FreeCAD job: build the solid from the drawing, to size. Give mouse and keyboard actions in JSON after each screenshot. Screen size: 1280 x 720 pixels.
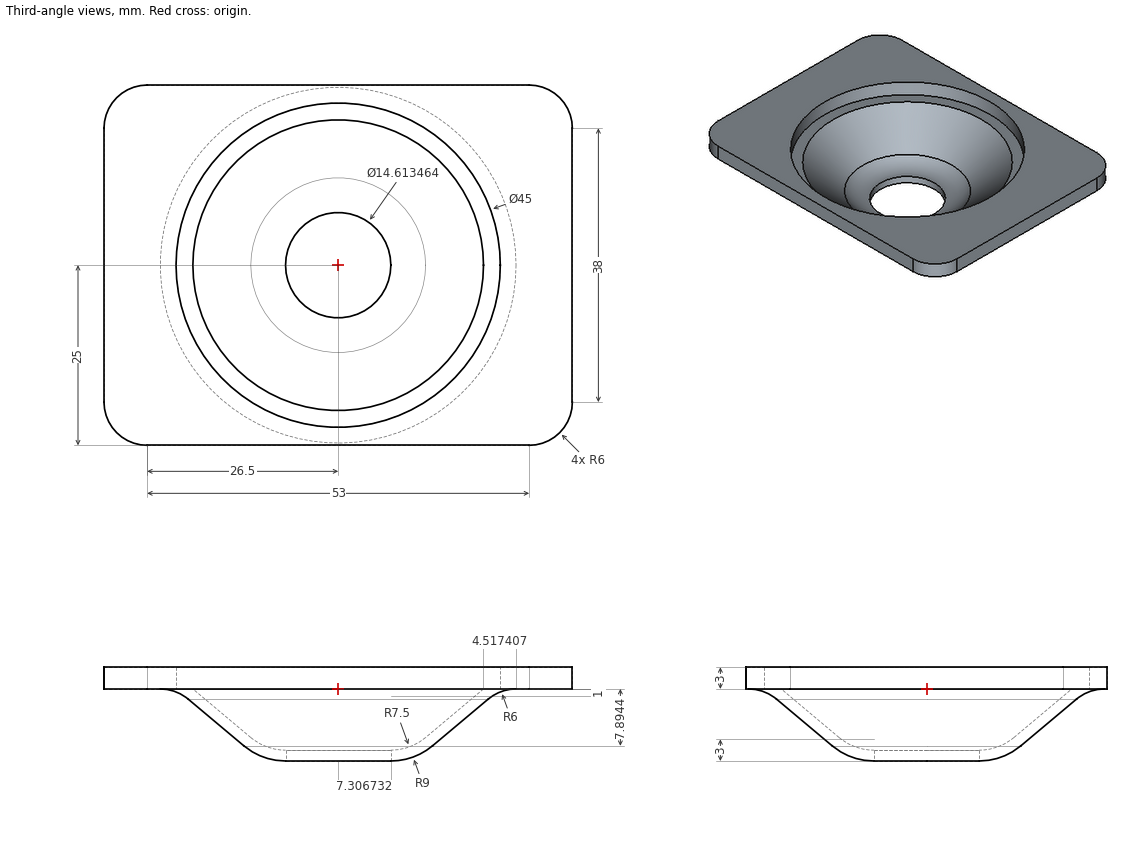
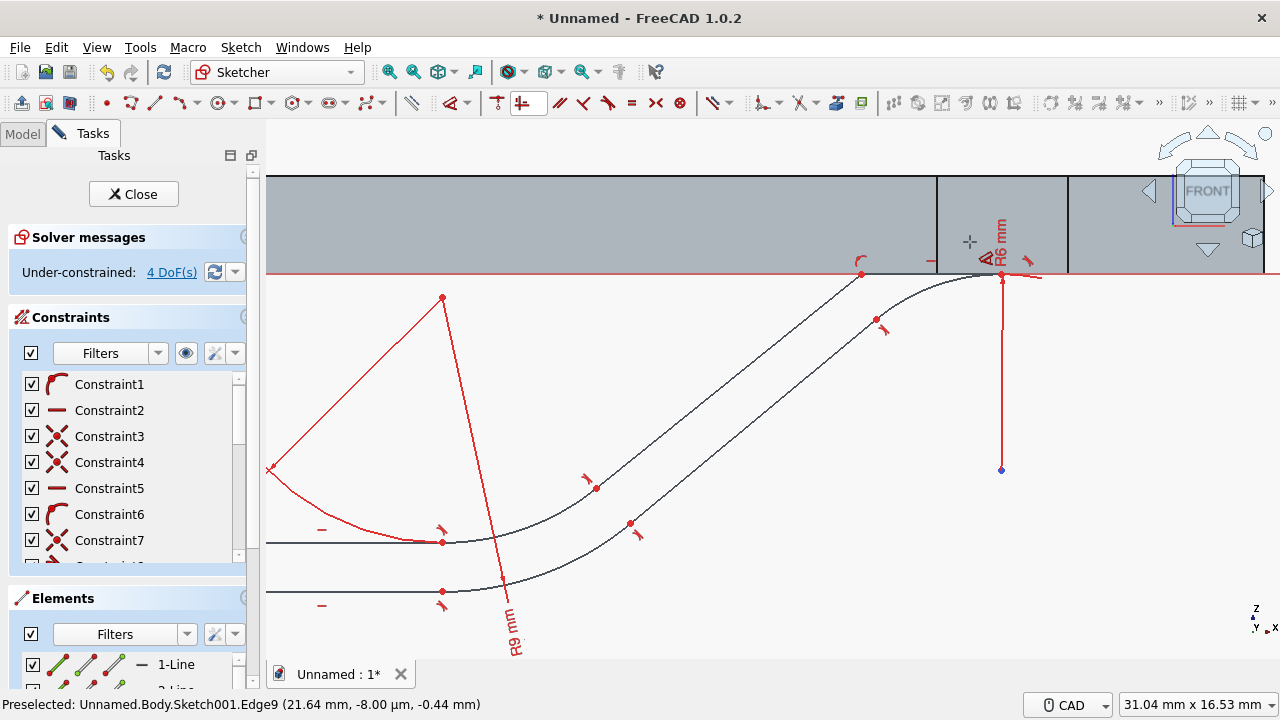
{"action": "left_click", "coordinate": [442, 298]}
{"action": "left_click", "coordinate": [476, 292]}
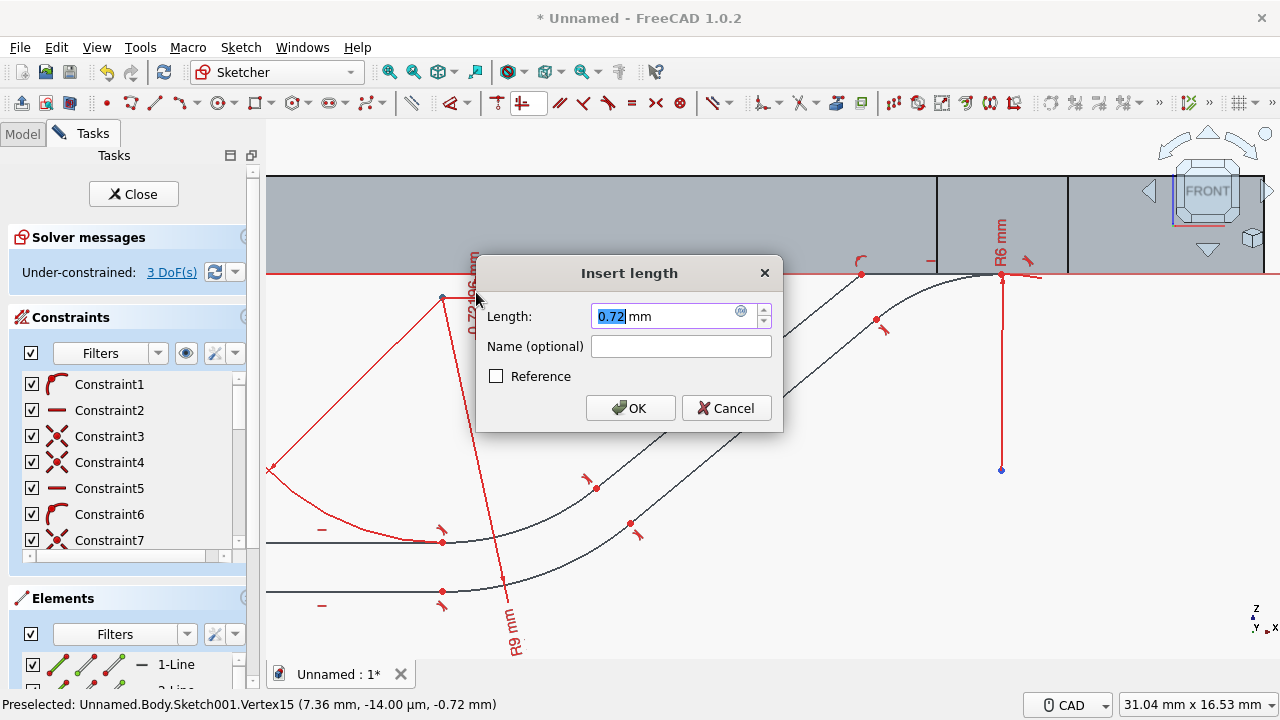
{"action": "type", "text": "1"}
{"action": "key", "text": "Return"}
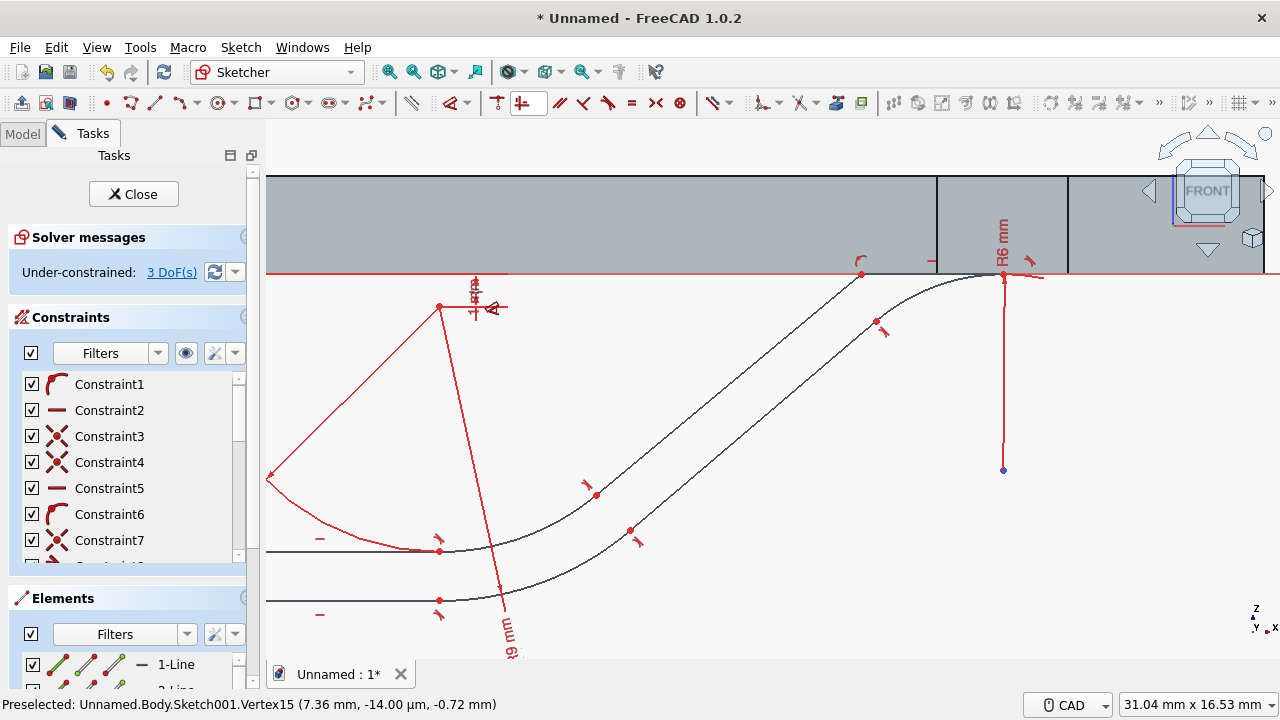
{"action": "left_click", "coordinate": [630, 531]}
{"action": "left_click", "coordinate": [664, 403]}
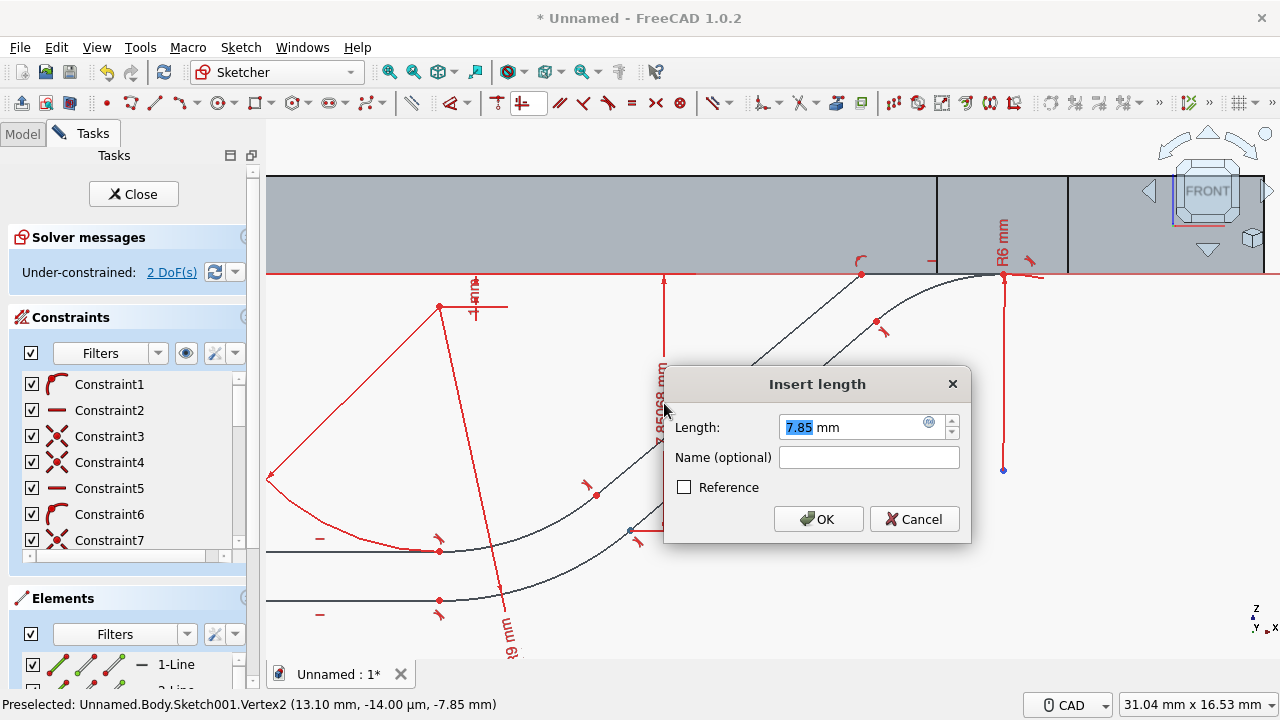
{"action": "type", "text": "7.8944"}
{"action": "key", "text": "Return"}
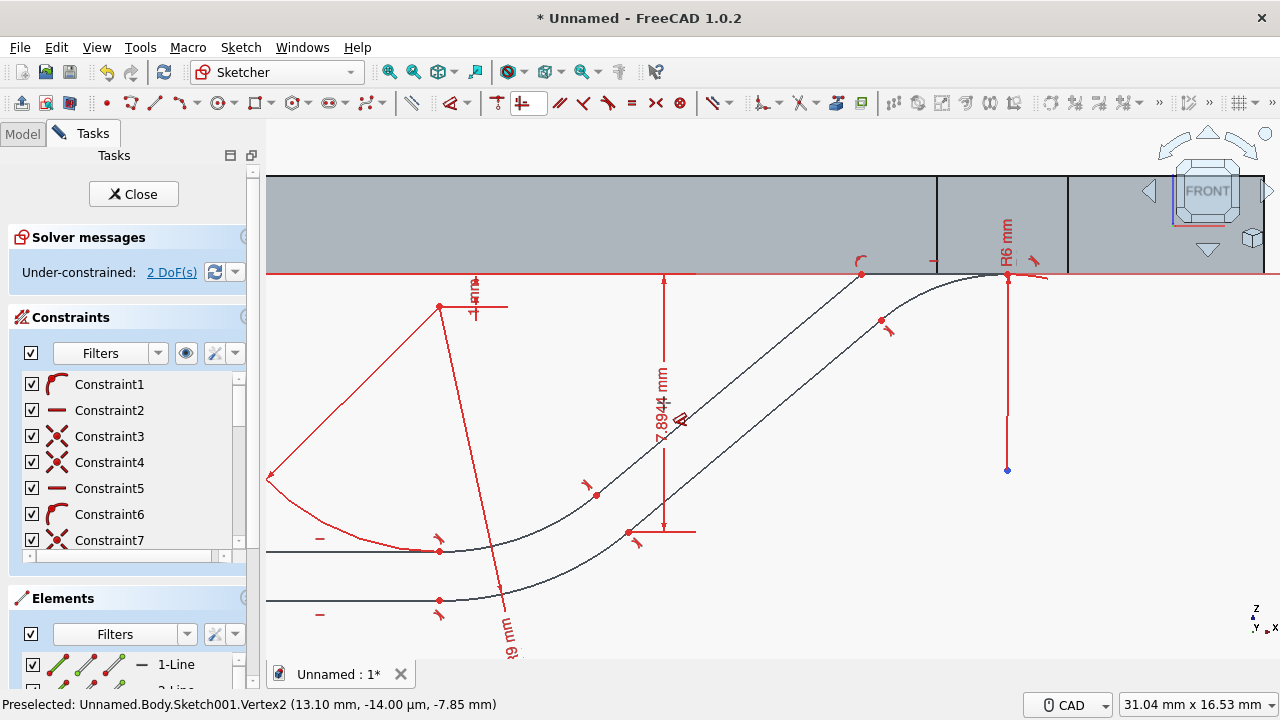
{"action": "left_click", "coordinate": [368, 601]}
{"action": "left_click", "coordinate": [367, 567]}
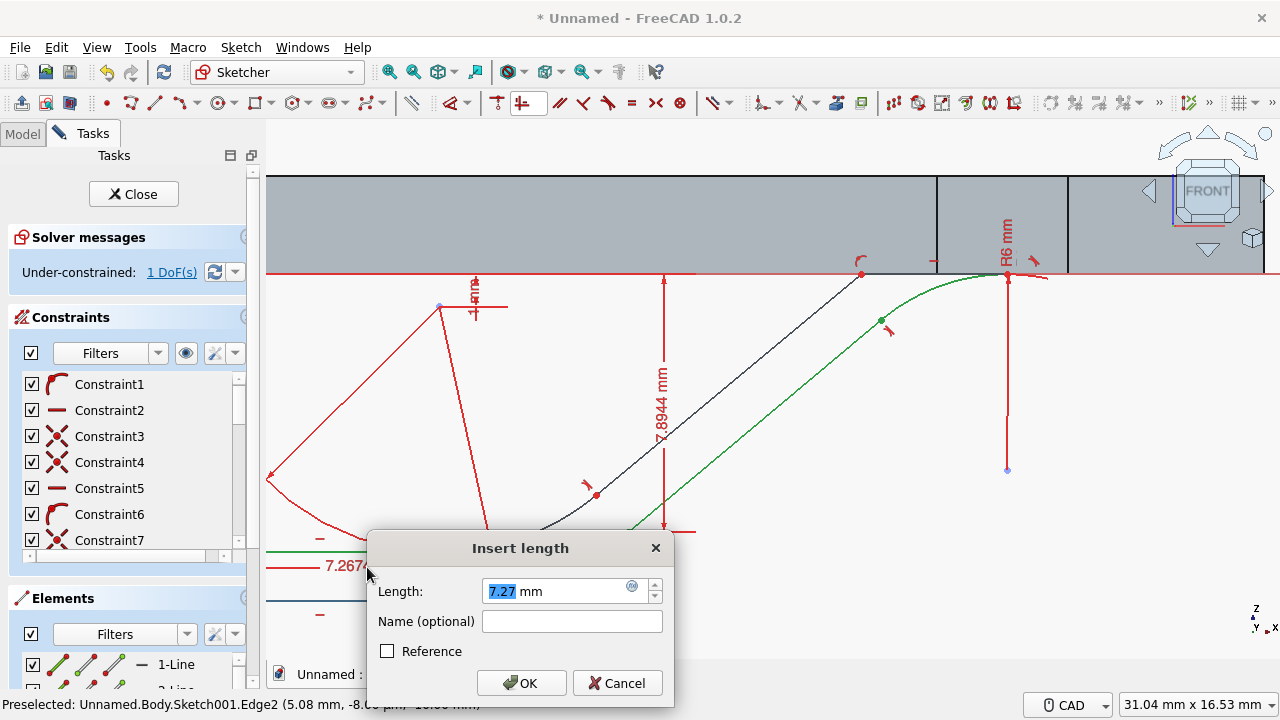
{"action": "type", "text": "7.306732"}
{"action": "key", "text": "Return"}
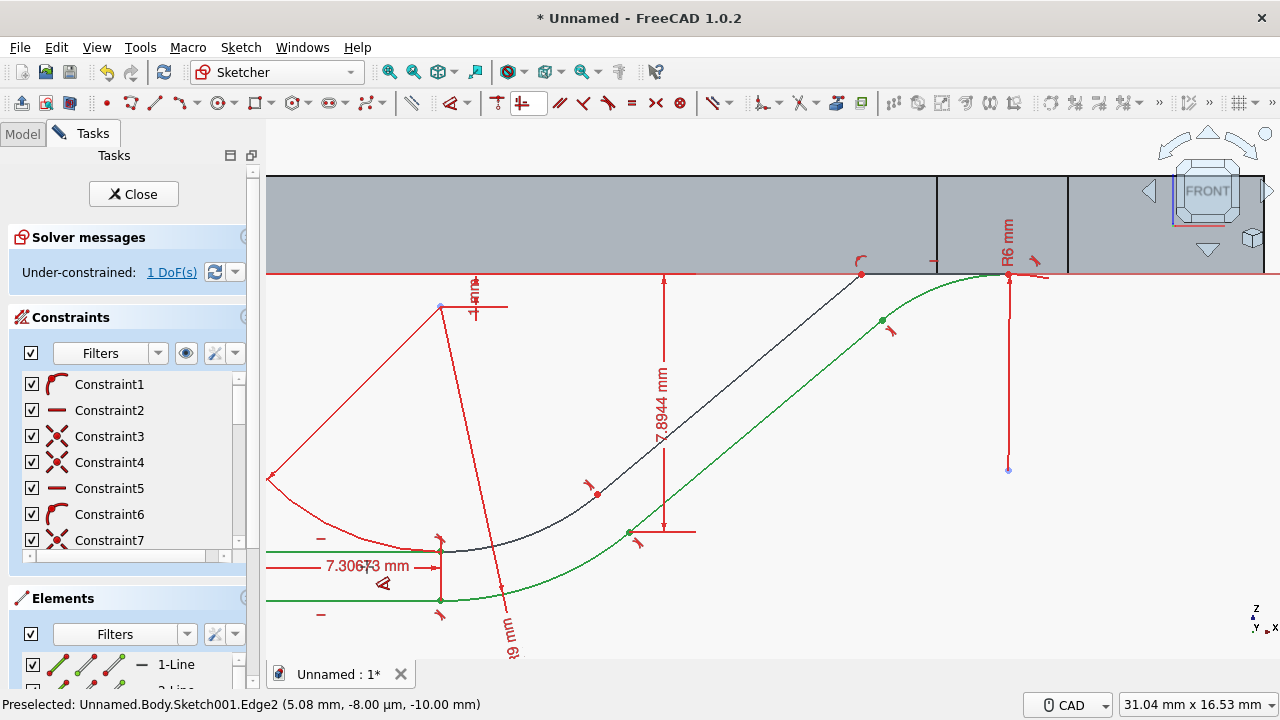
{"action": "left_click", "coordinate": [906, 274]}
{"action": "left_click", "coordinate": [884, 240]}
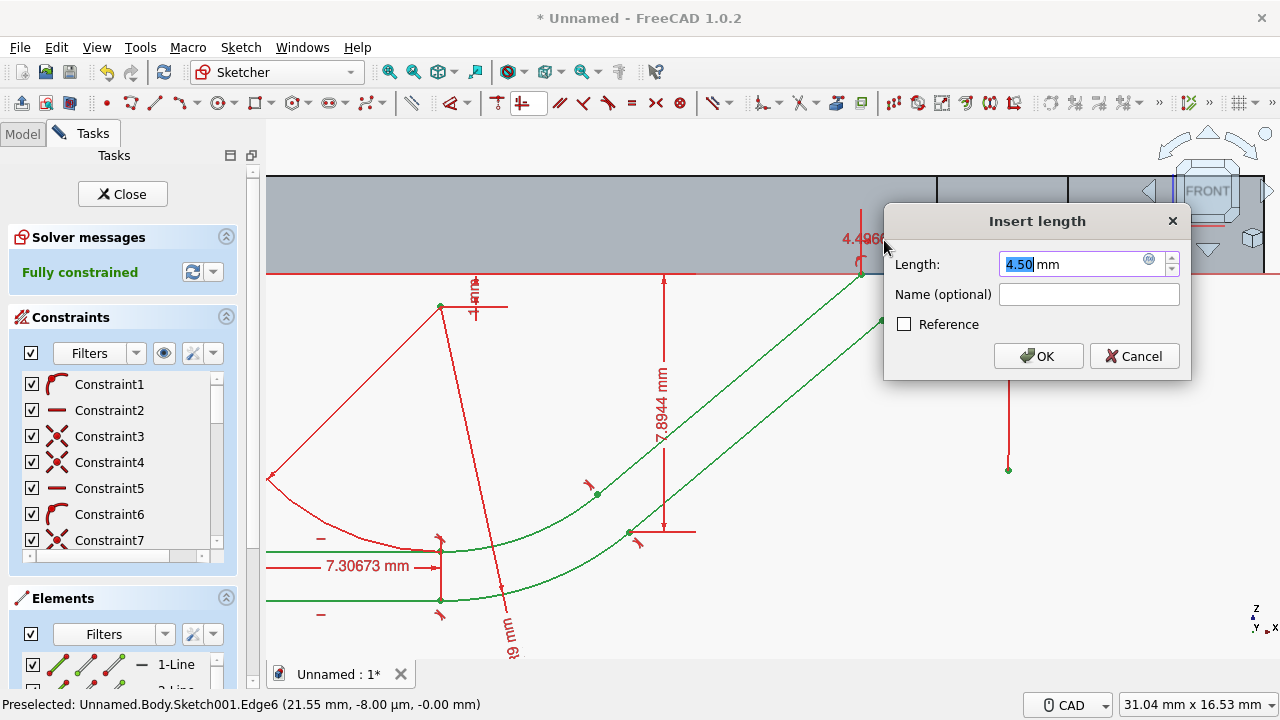
{"action": "type", "text": "4.517407"}
{"action": "key", "text": "Return"}
{"action": "key", "text": "Escape"}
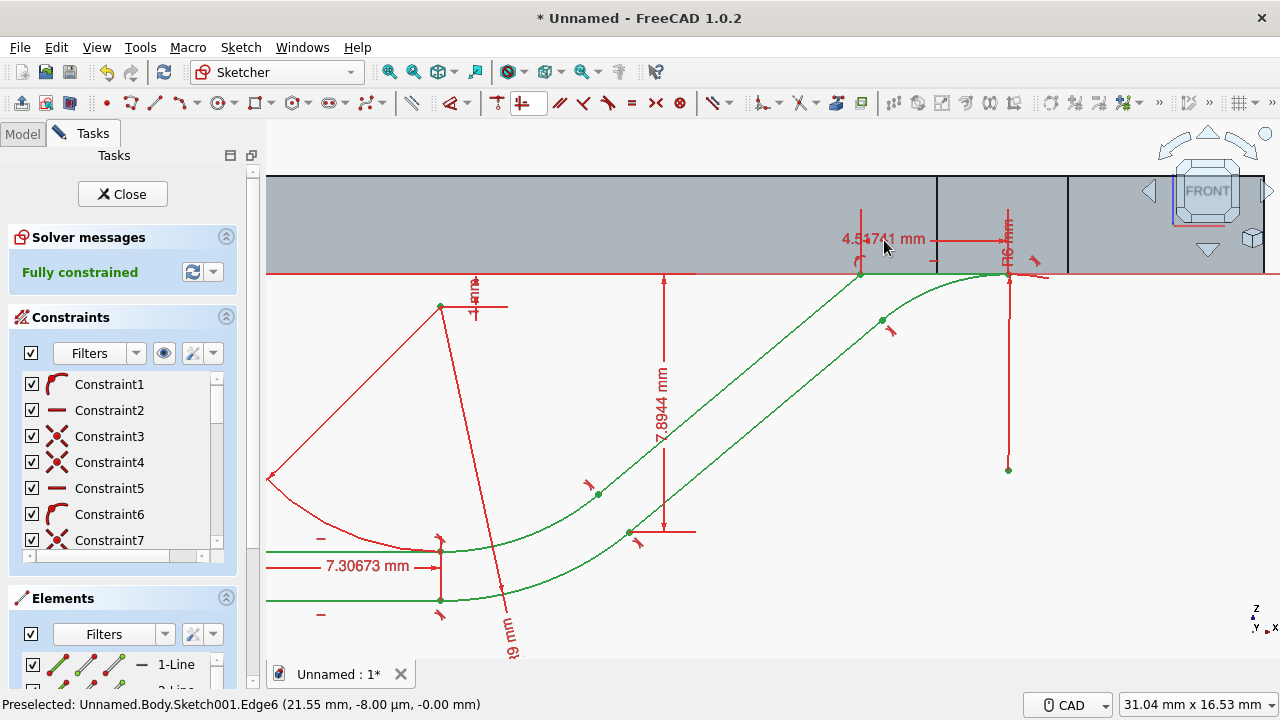
{"action": "left_click", "coordinate": [123, 194]}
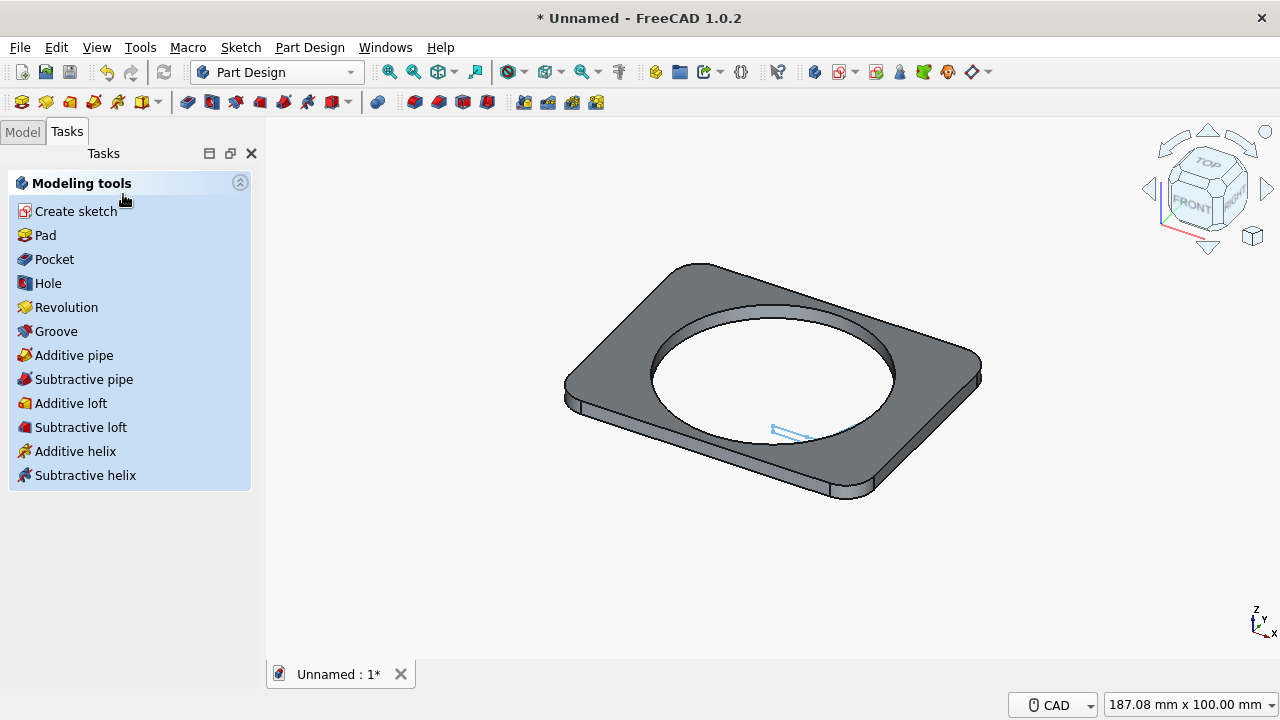
{"action": "left_click", "coordinate": [46, 102]}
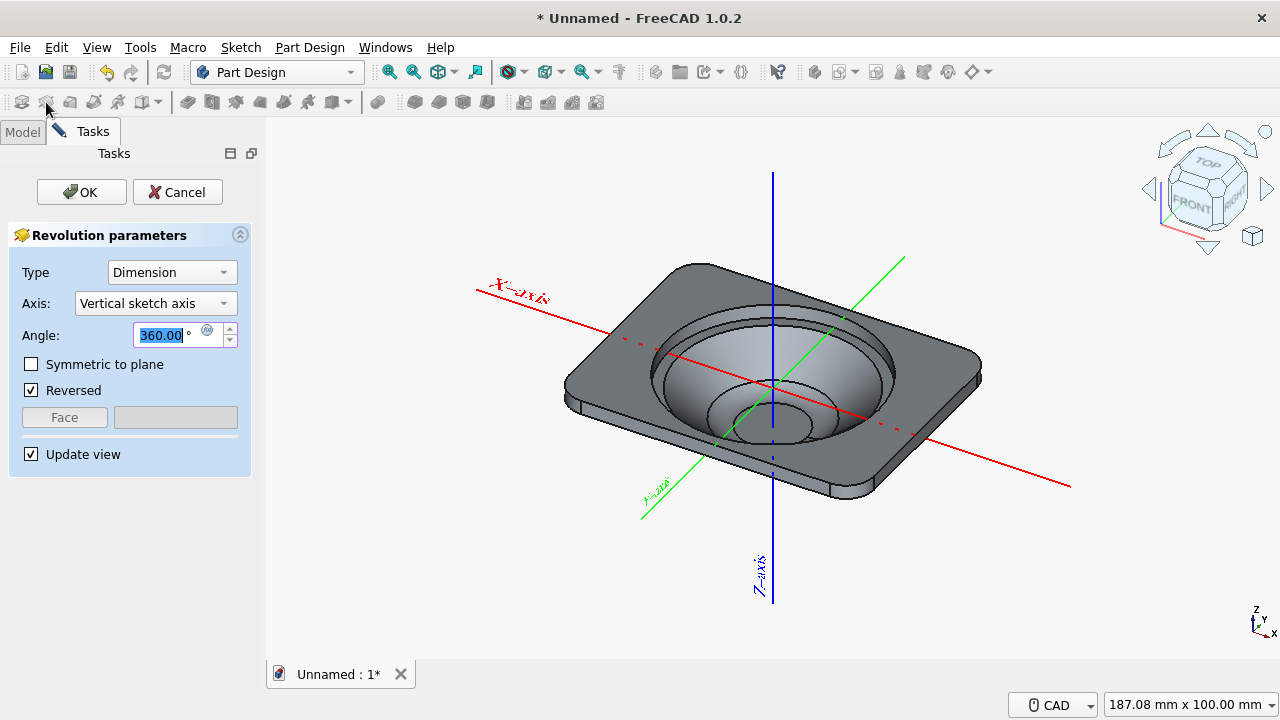
{"action": "left_click", "coordinate": [82, 192]}